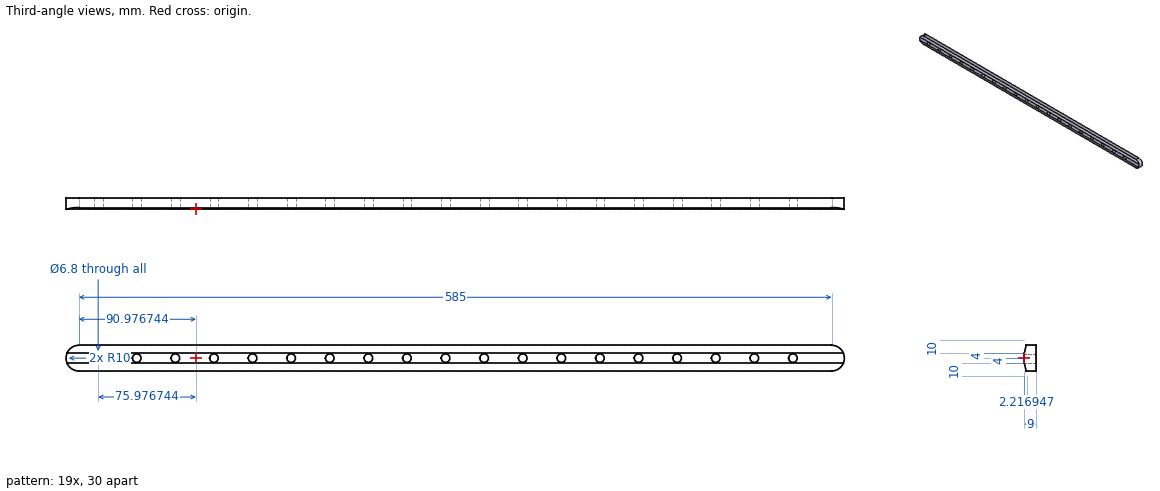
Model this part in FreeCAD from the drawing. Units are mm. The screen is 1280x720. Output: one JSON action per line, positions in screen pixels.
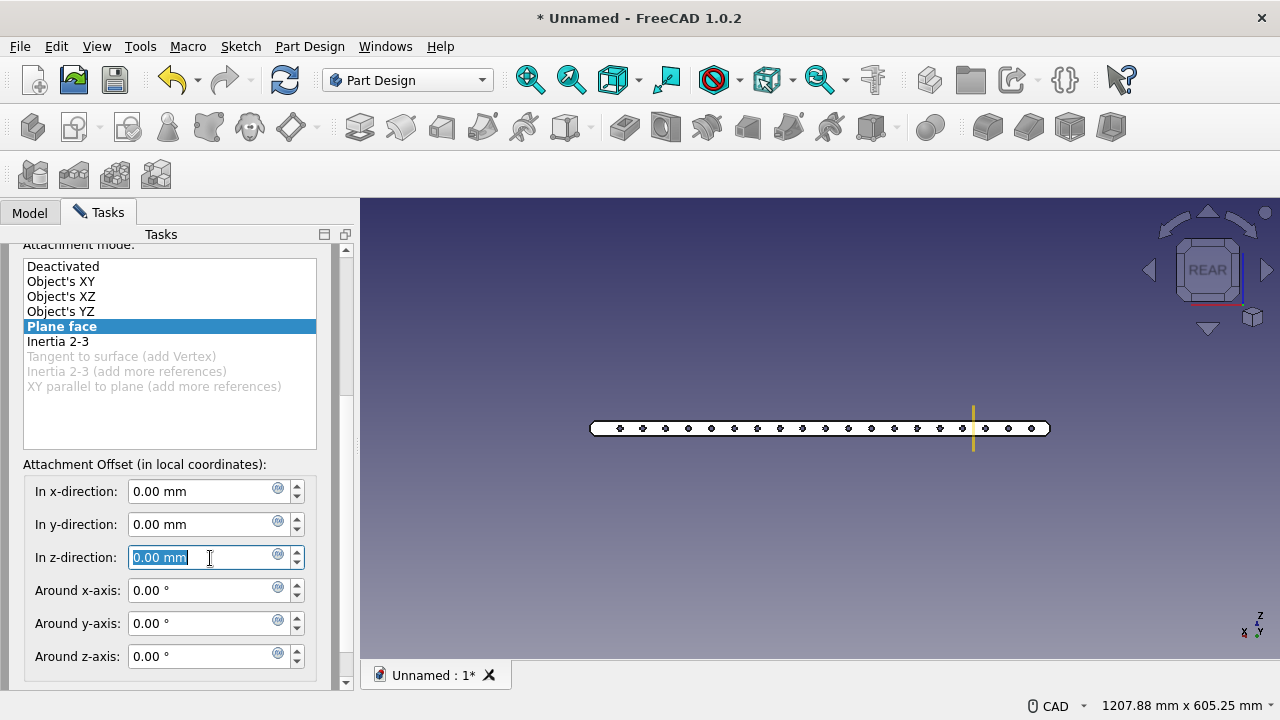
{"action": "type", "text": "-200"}
{"action": "key", "text": "Tab"}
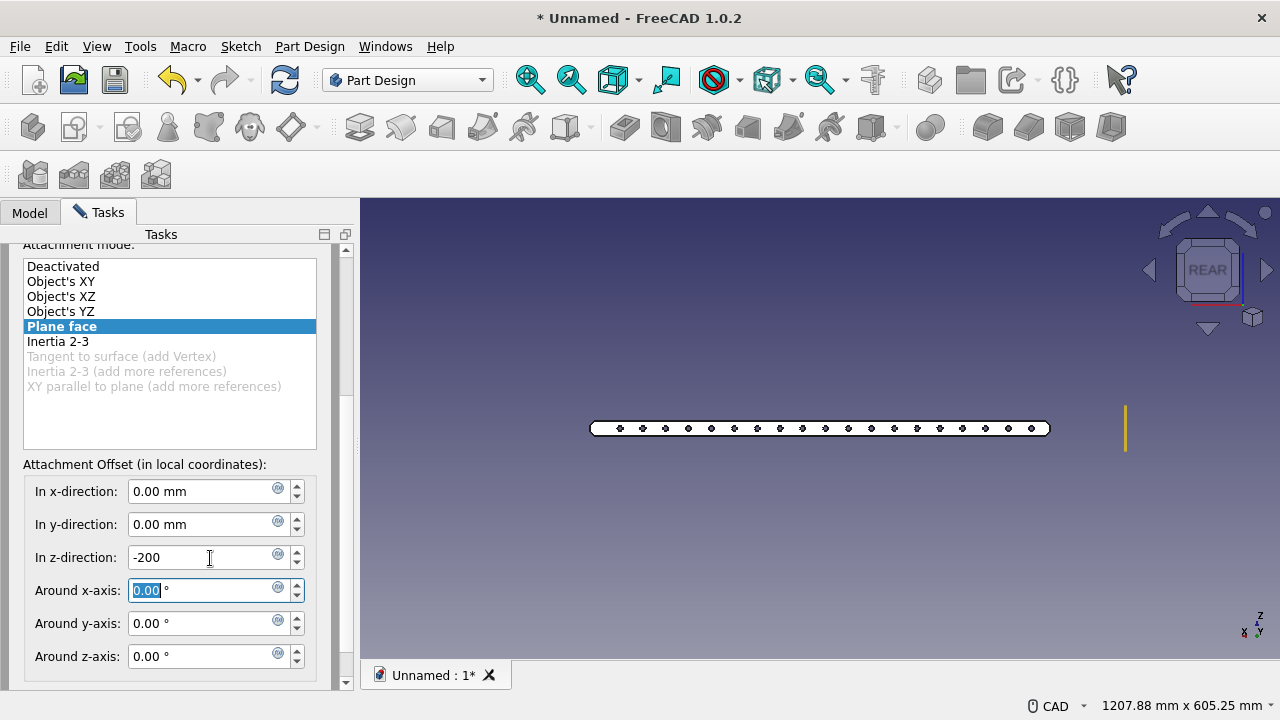
{"action": "scroll", "coordinate": [346, 467], "scroll_direction": "up", "scroll_amount": 5}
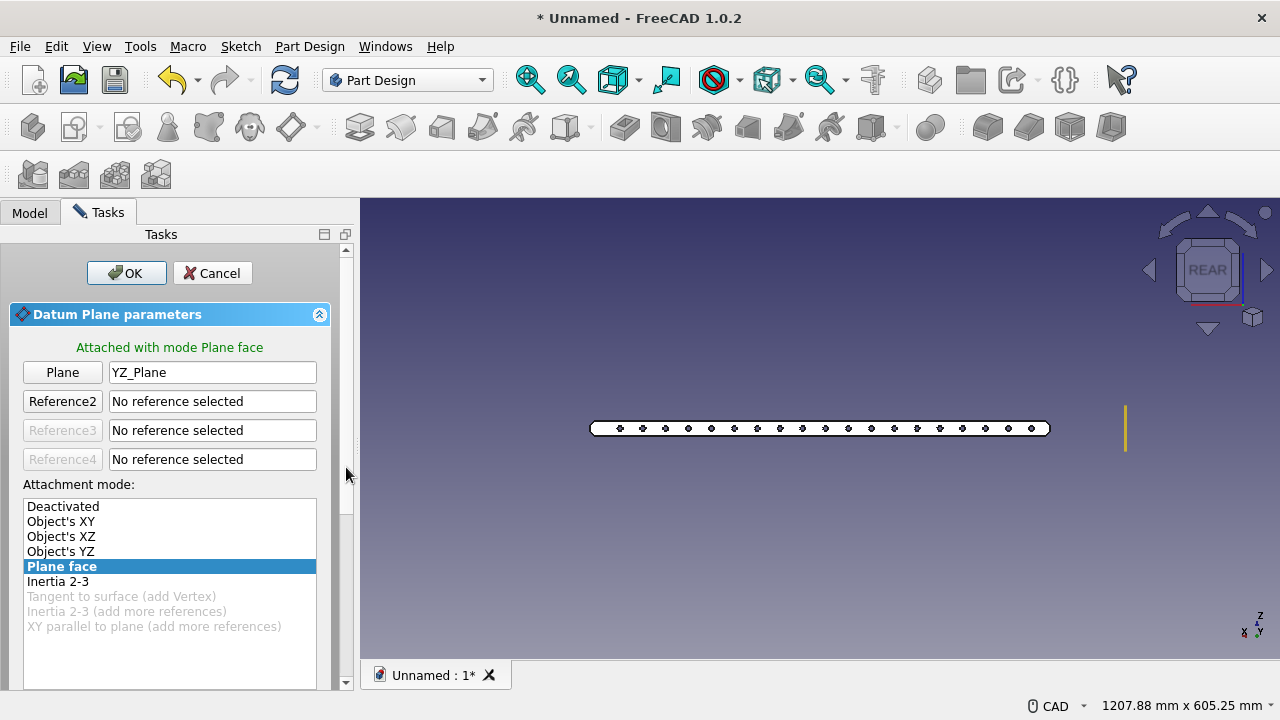
{"action": "left_click", "coordinate": [127, 273]}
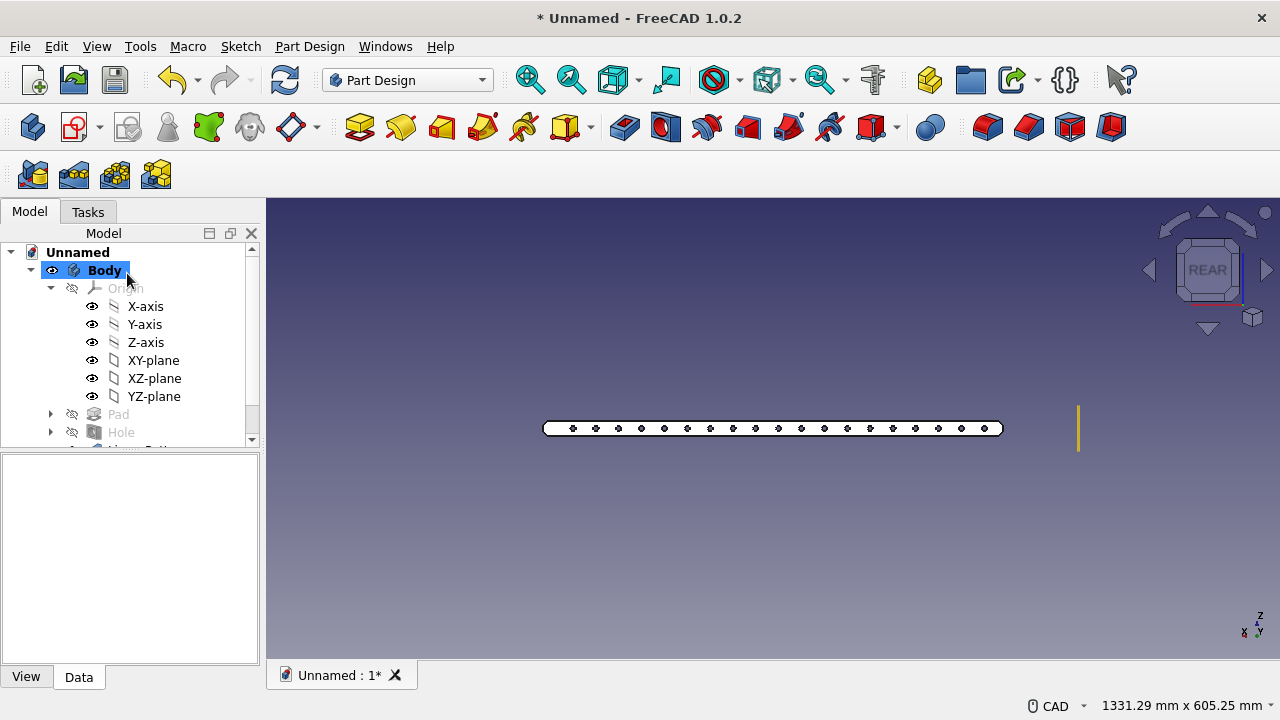
{"action": "scroll", "coordinate": [101, 338], "scroll_direction": "down", "scroll_amount": 3}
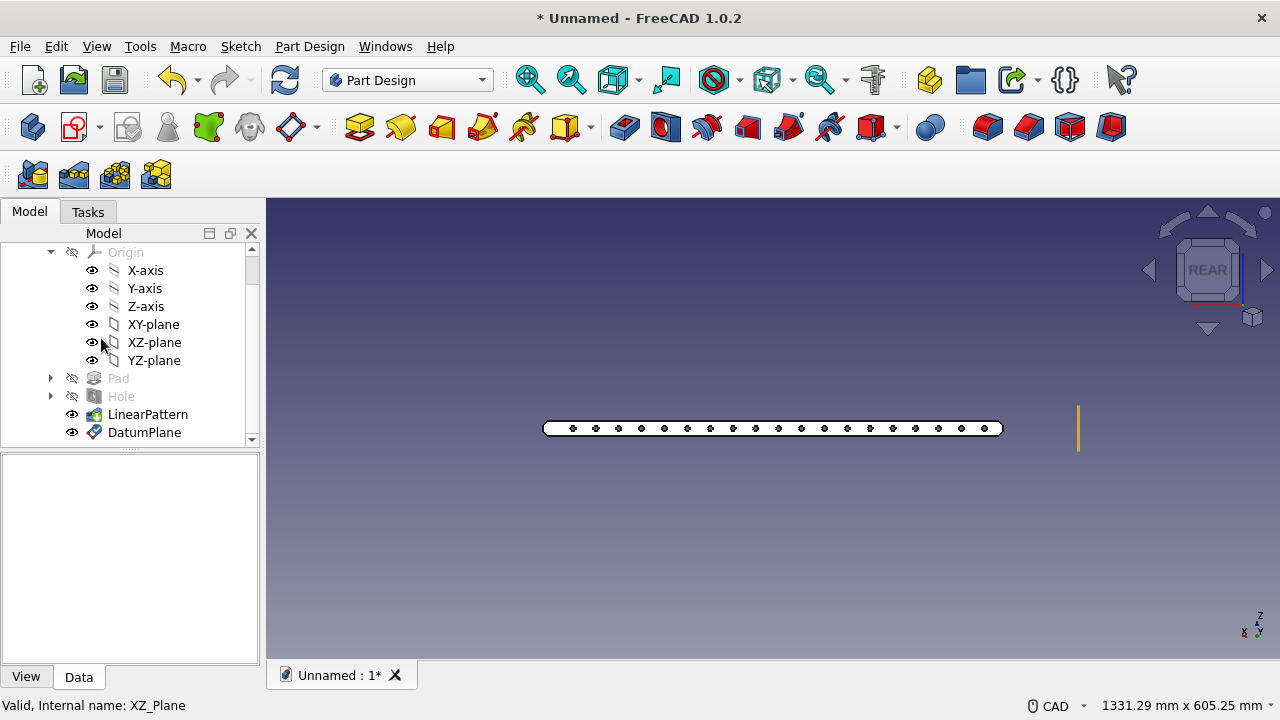
{"action": "left_click", "coordinate": [117, 432]}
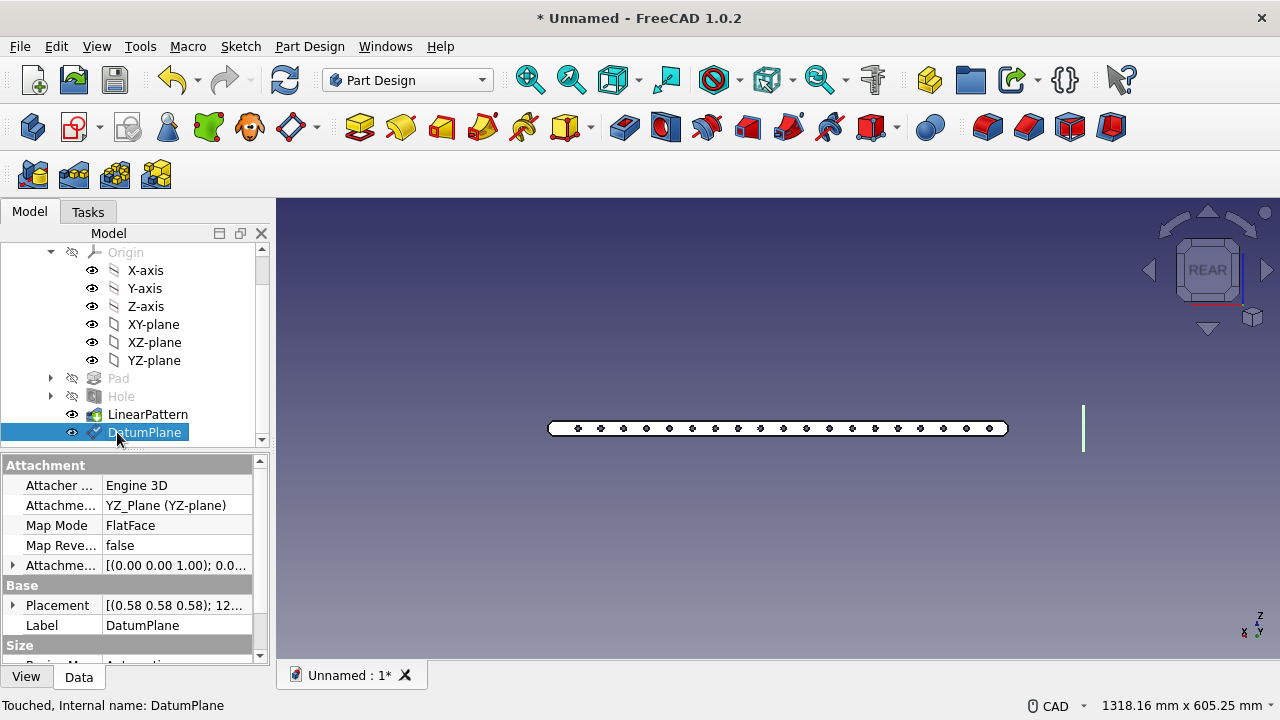
{"action": "left_click", "coordinate": [74, 128]}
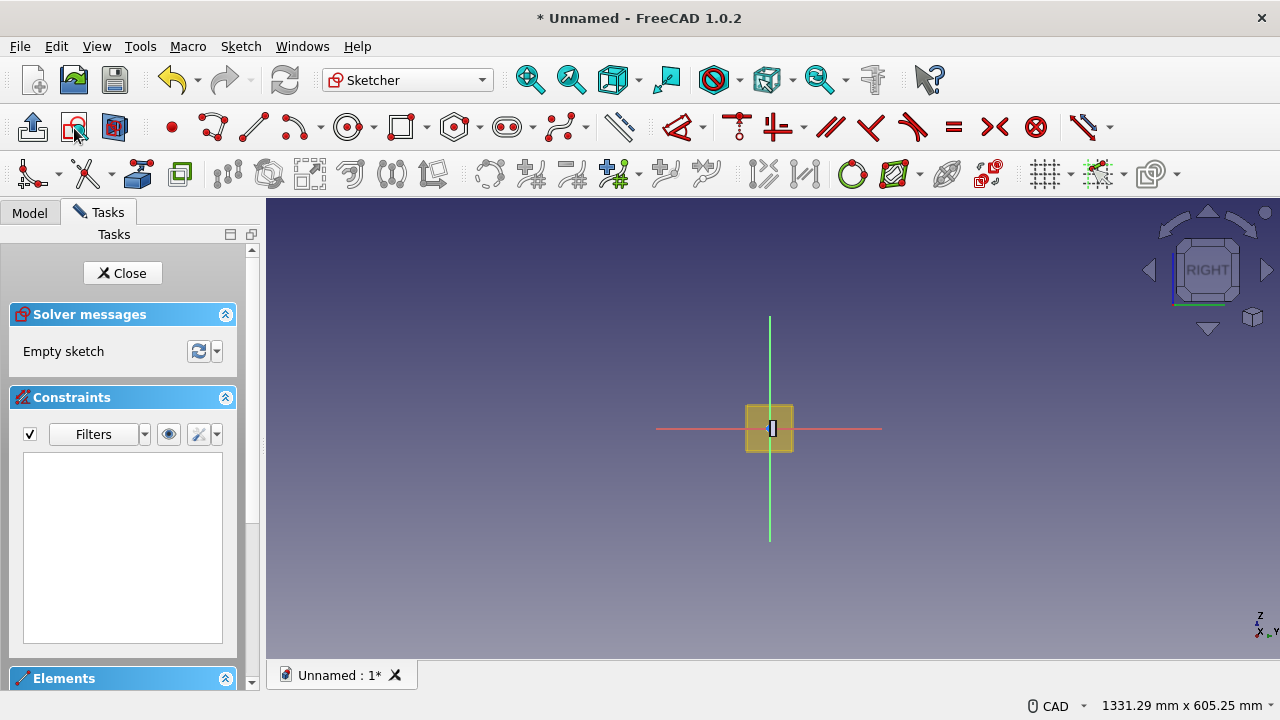
{"action": "left_click", "coordinate": [115, 128]}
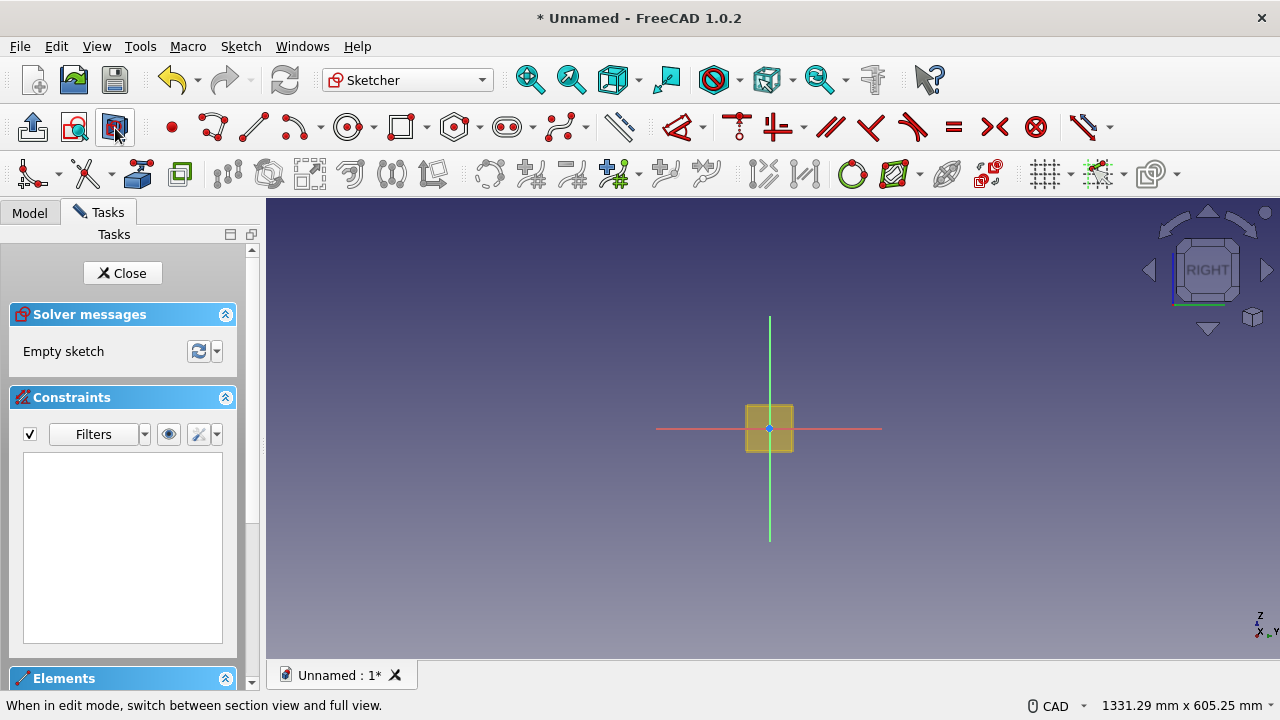
{"action": "scroll", "coordinate": [776, 429], "scroll_direction": "up", "scroll_amount": 13}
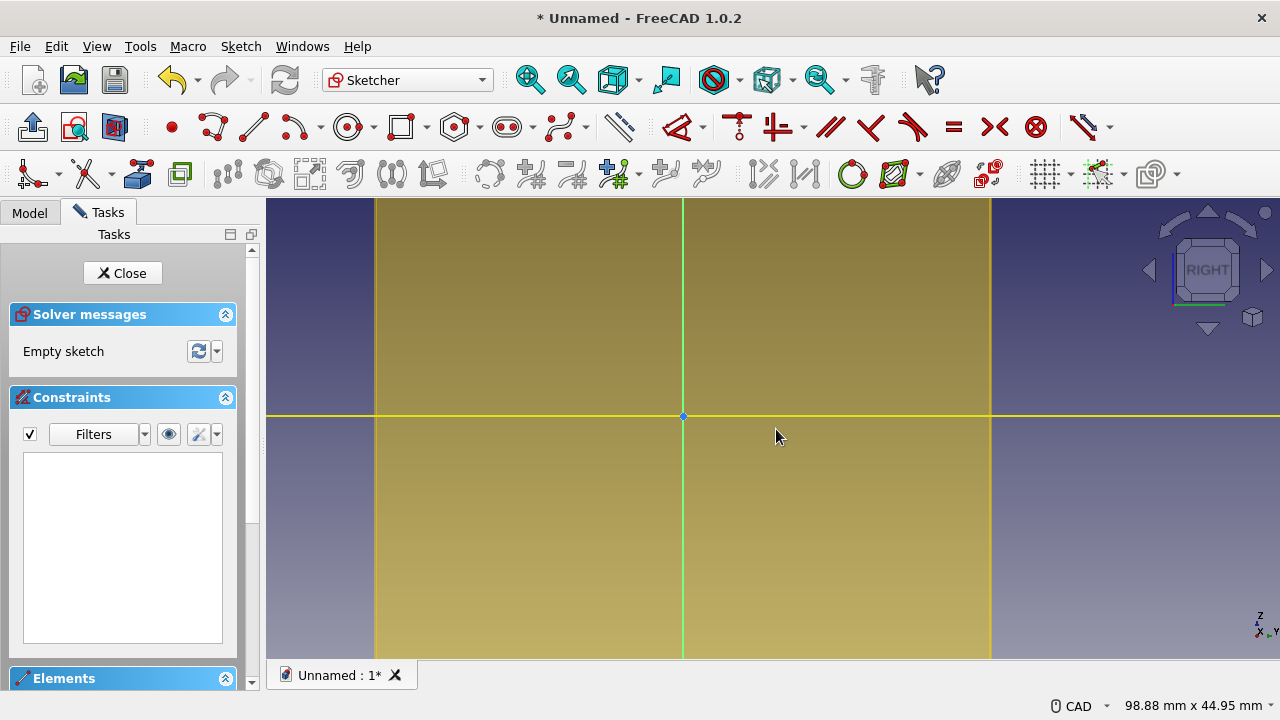
{"action": "left_click", "coordinate": [213, 128]}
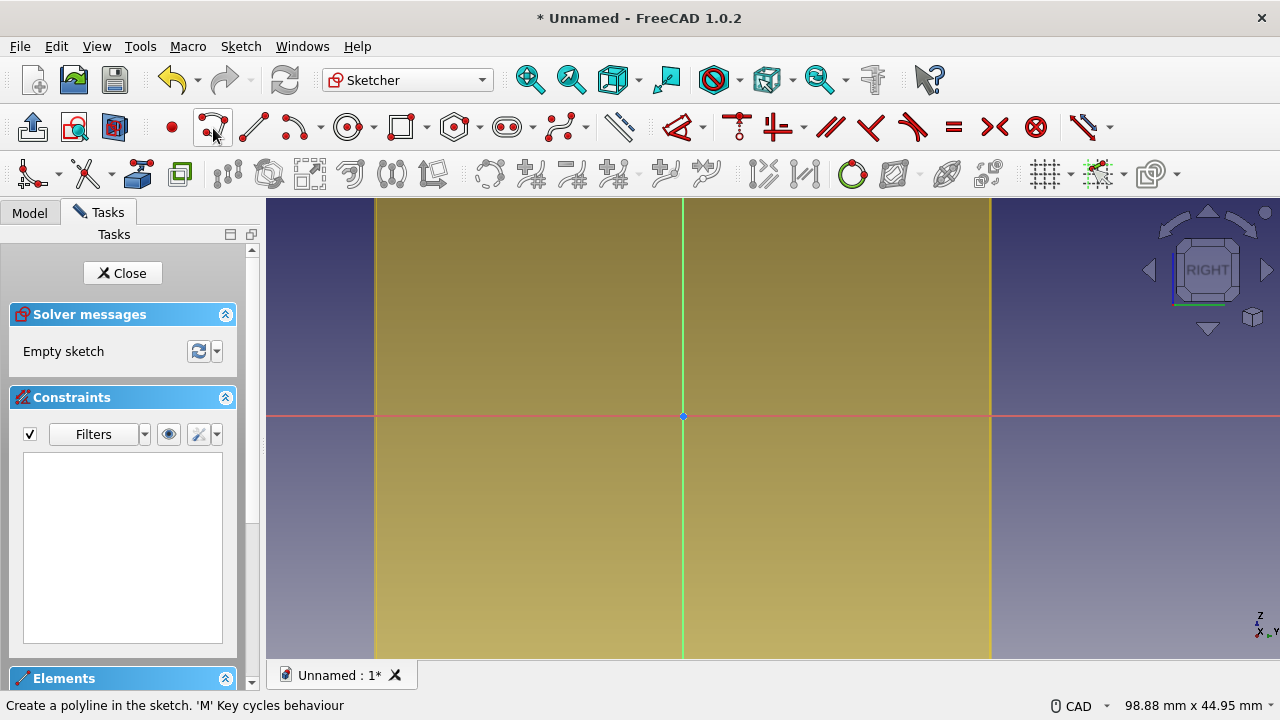
{"action": "left_click", "coordinate": [683, 457]}
{"action": "left_click", "coordinate": [692, 560]}
{"action": "left_click", "coordinate": [706, 560]}
{"action": "left_click", "coordinate": [683, 458]}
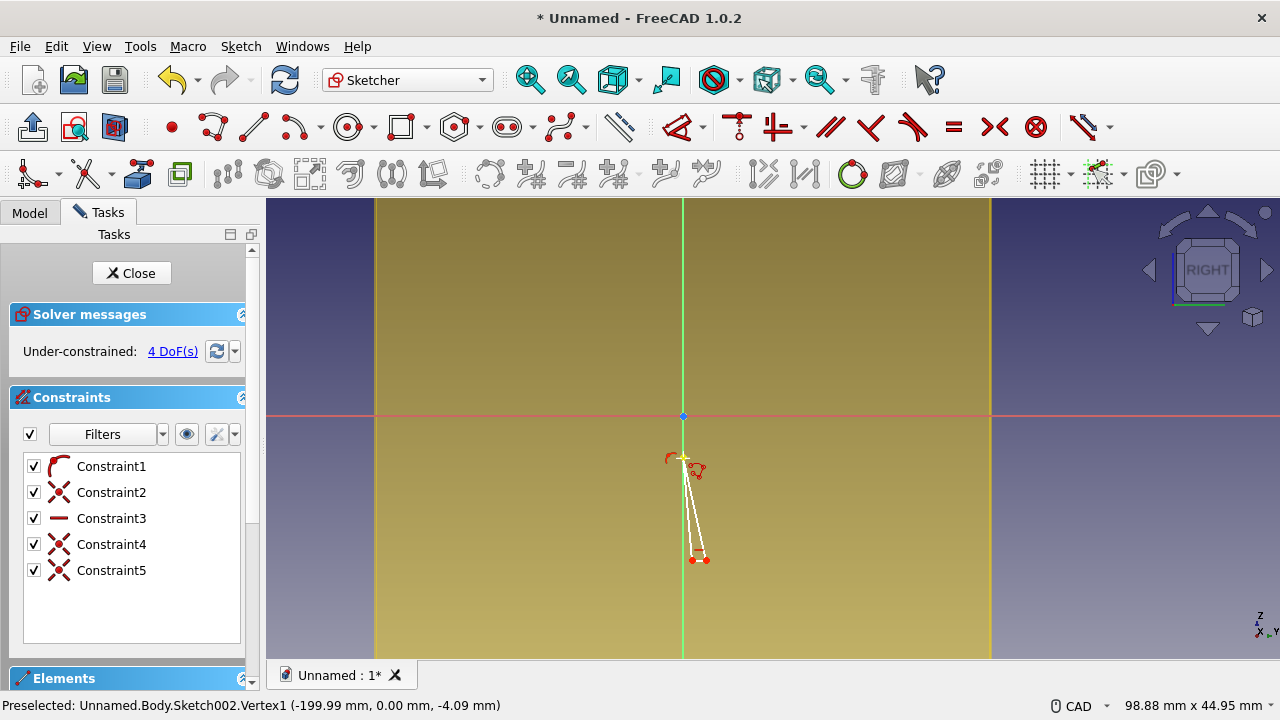
{"action": "left_click", "coordinate": [683, 375]}
{"action": "left_click", "coordinate": [706, 272]}
{"action": "left_click", "coordinate": [692, 272]}
{"action": "left_click", "coordinate": [683, 376]}
{"action": "key", "text": "Escape"}
{"action": "key", "text": "Escape"}